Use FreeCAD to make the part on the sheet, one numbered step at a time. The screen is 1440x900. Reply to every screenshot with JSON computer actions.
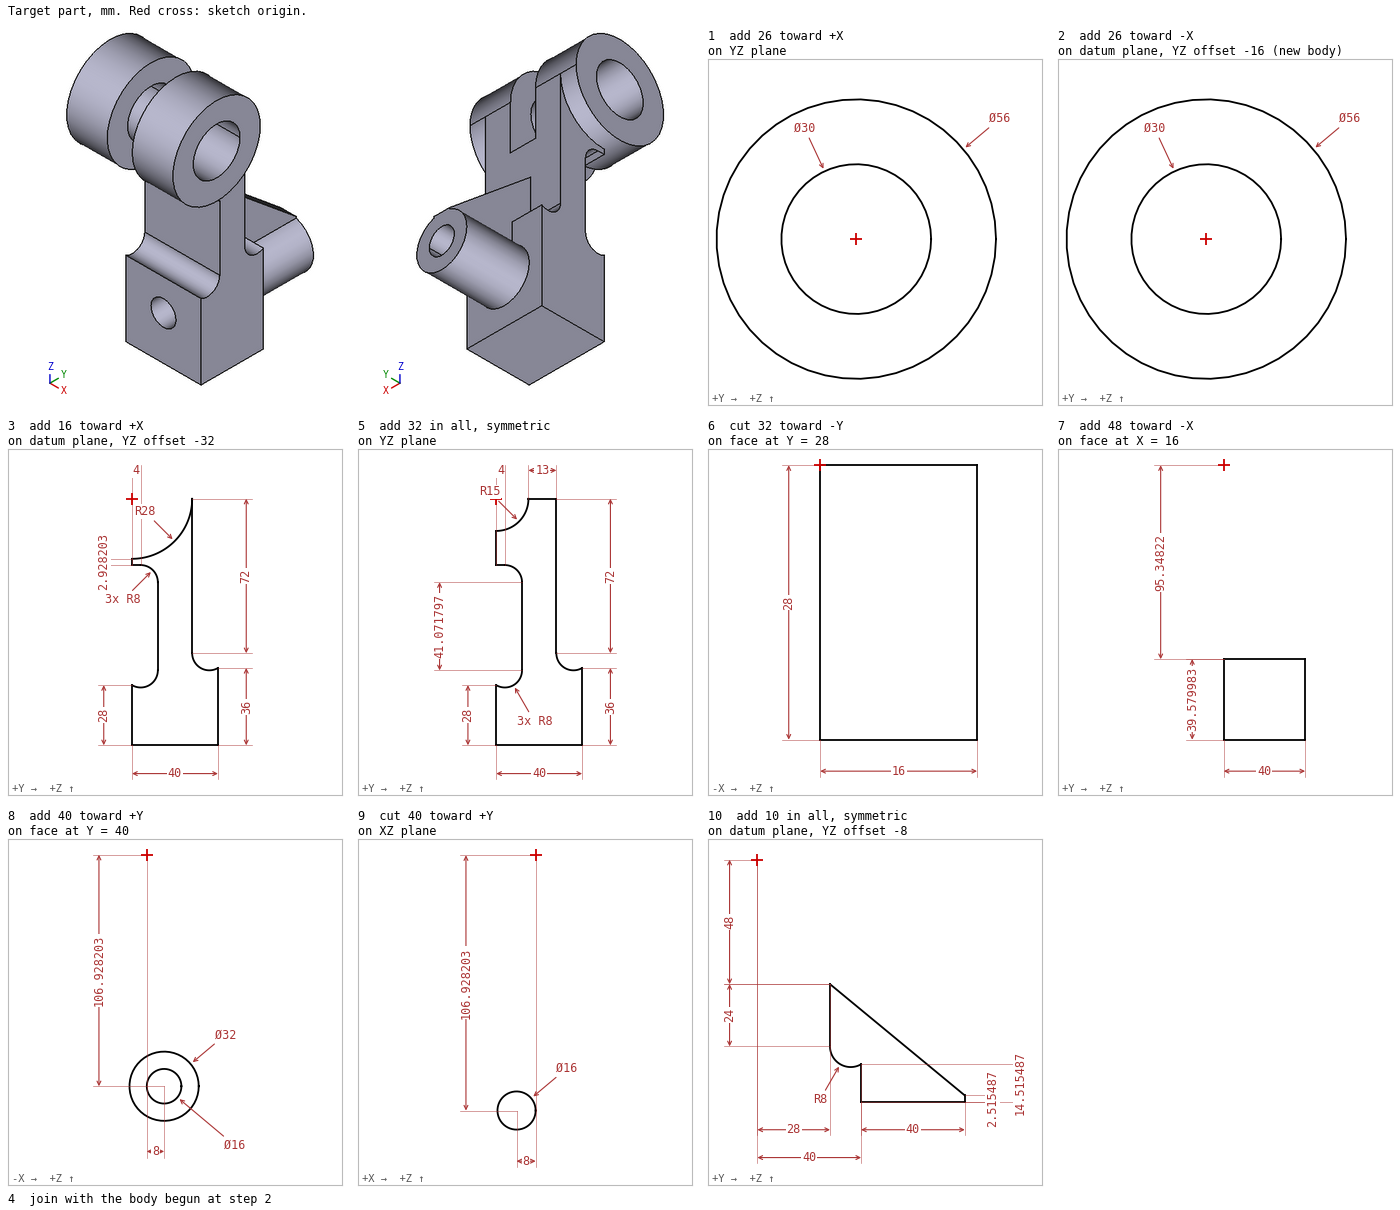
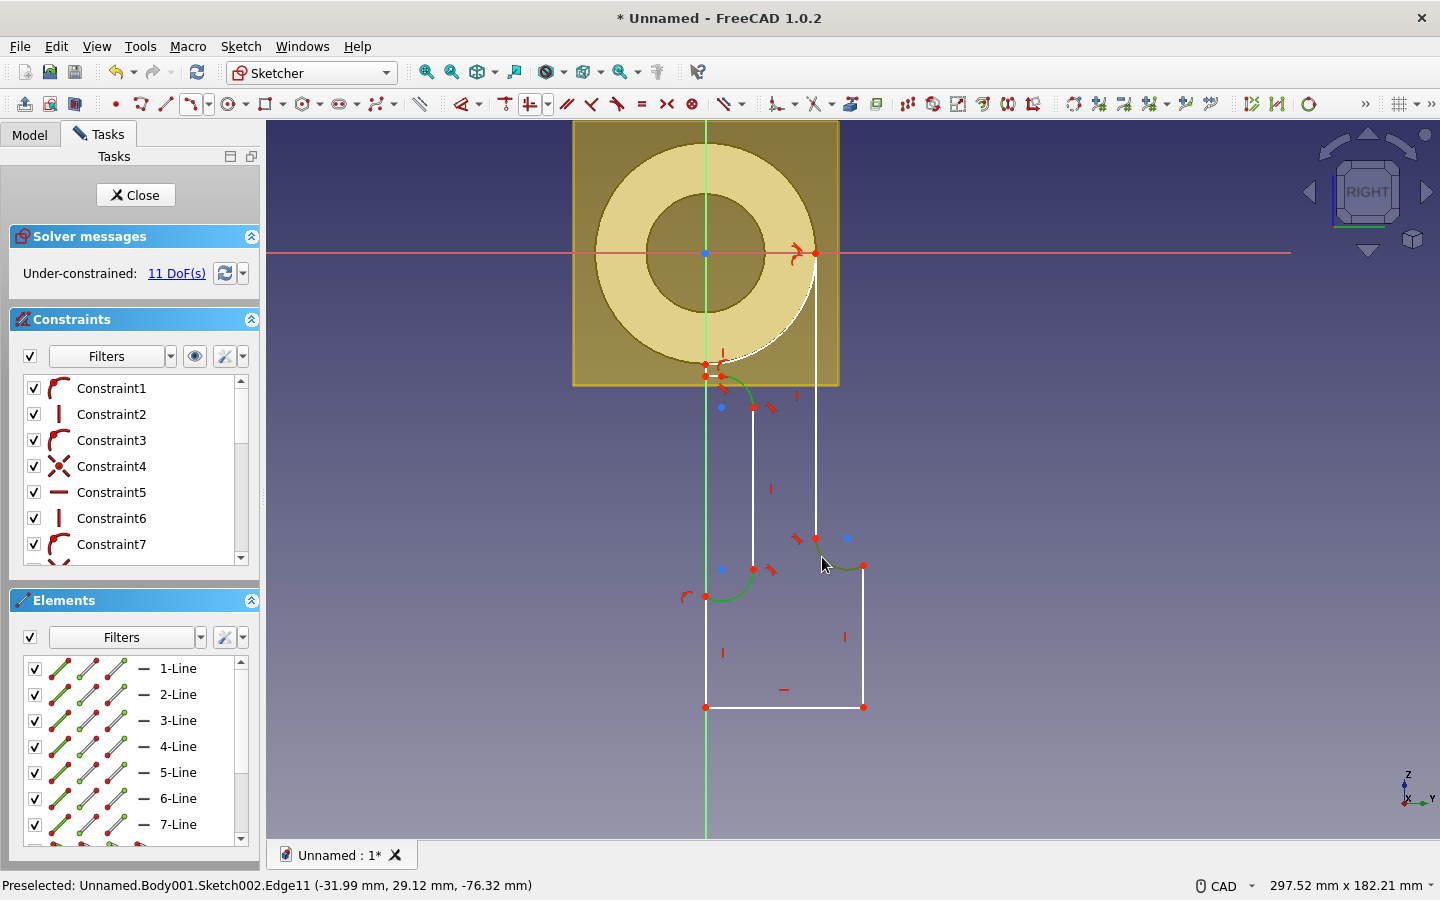
{"action": "key", "text": "e"}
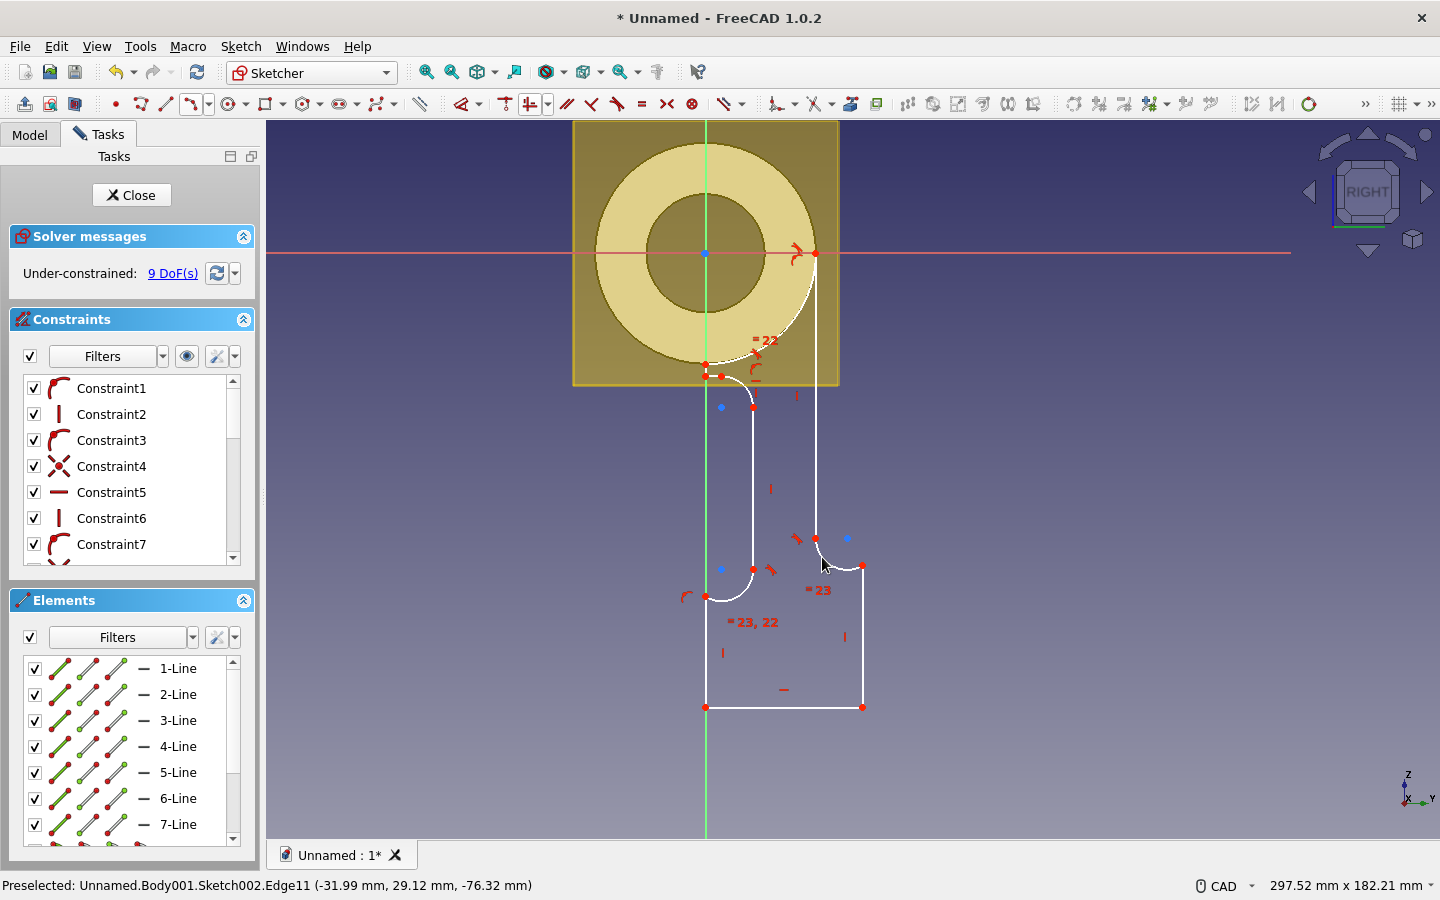
{"action": "left_click", "coordinate": [705, 253]}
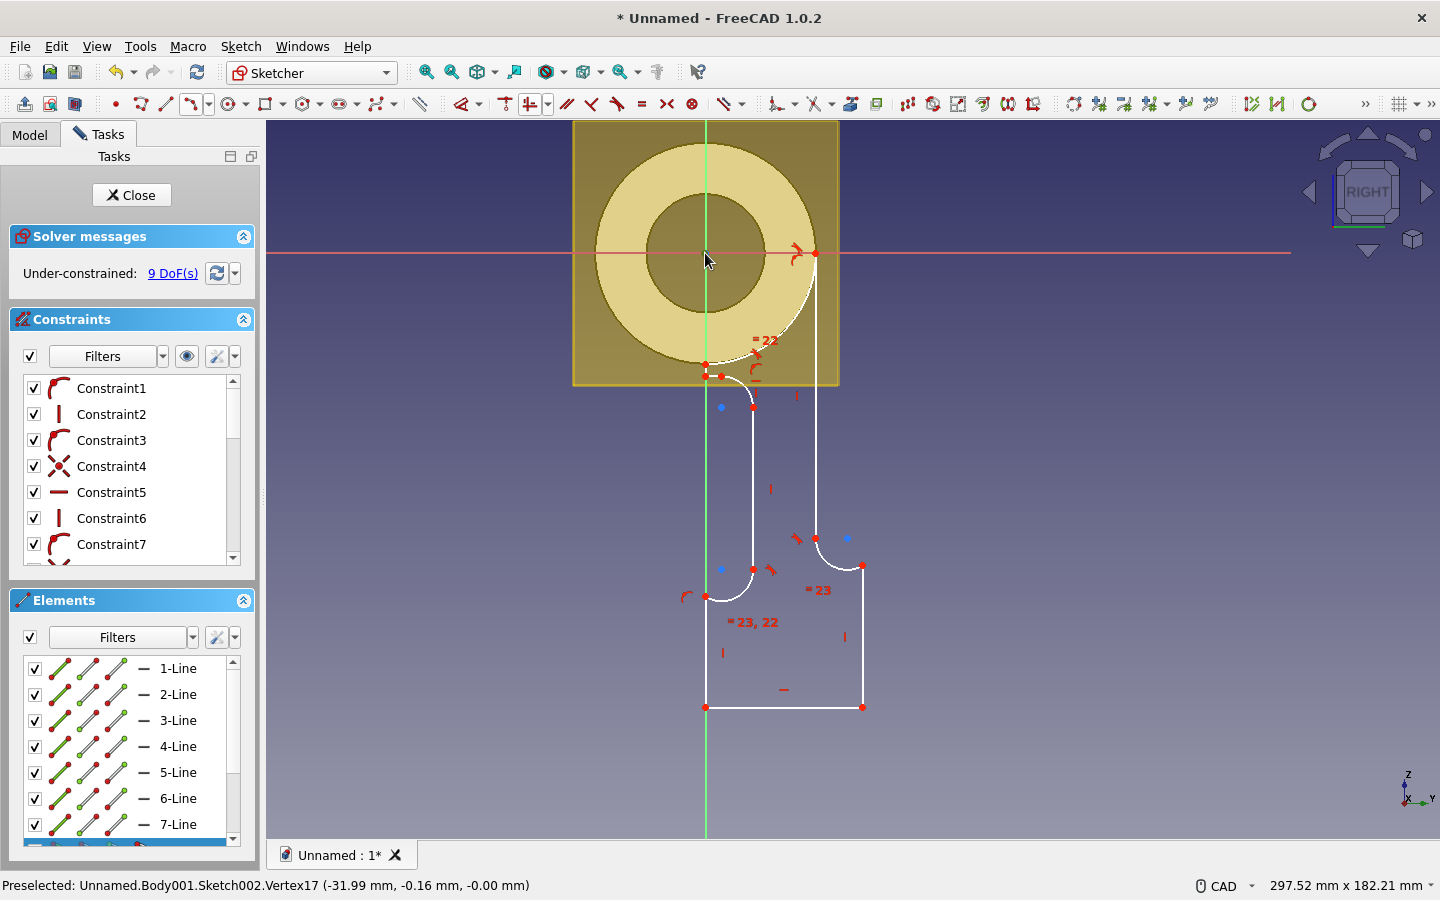
{"action": "left_click", "coordinate": [706, 764]}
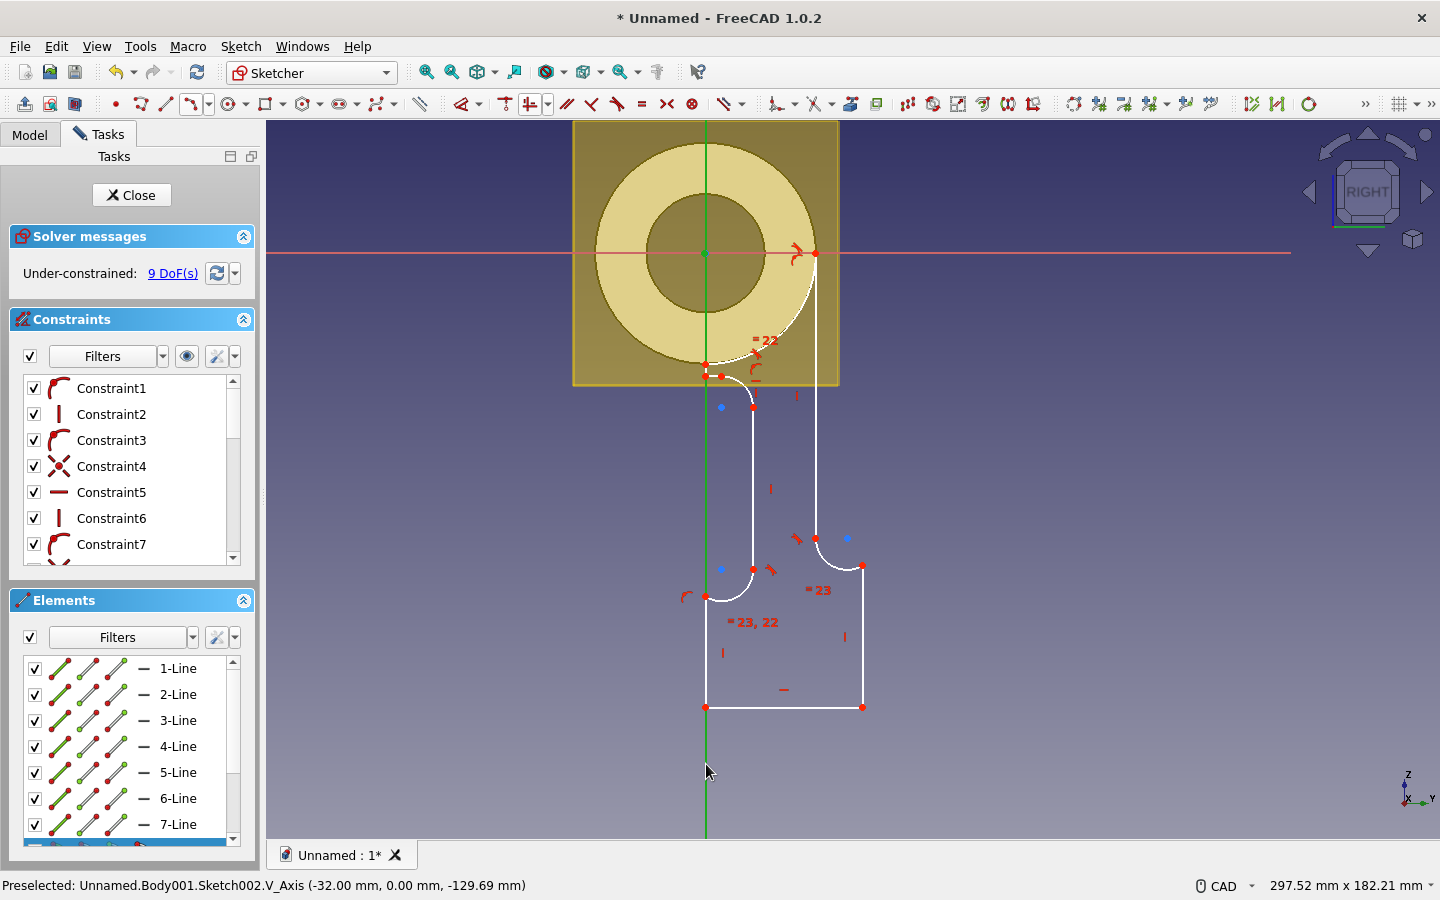
{"action": "key", "text": "c"}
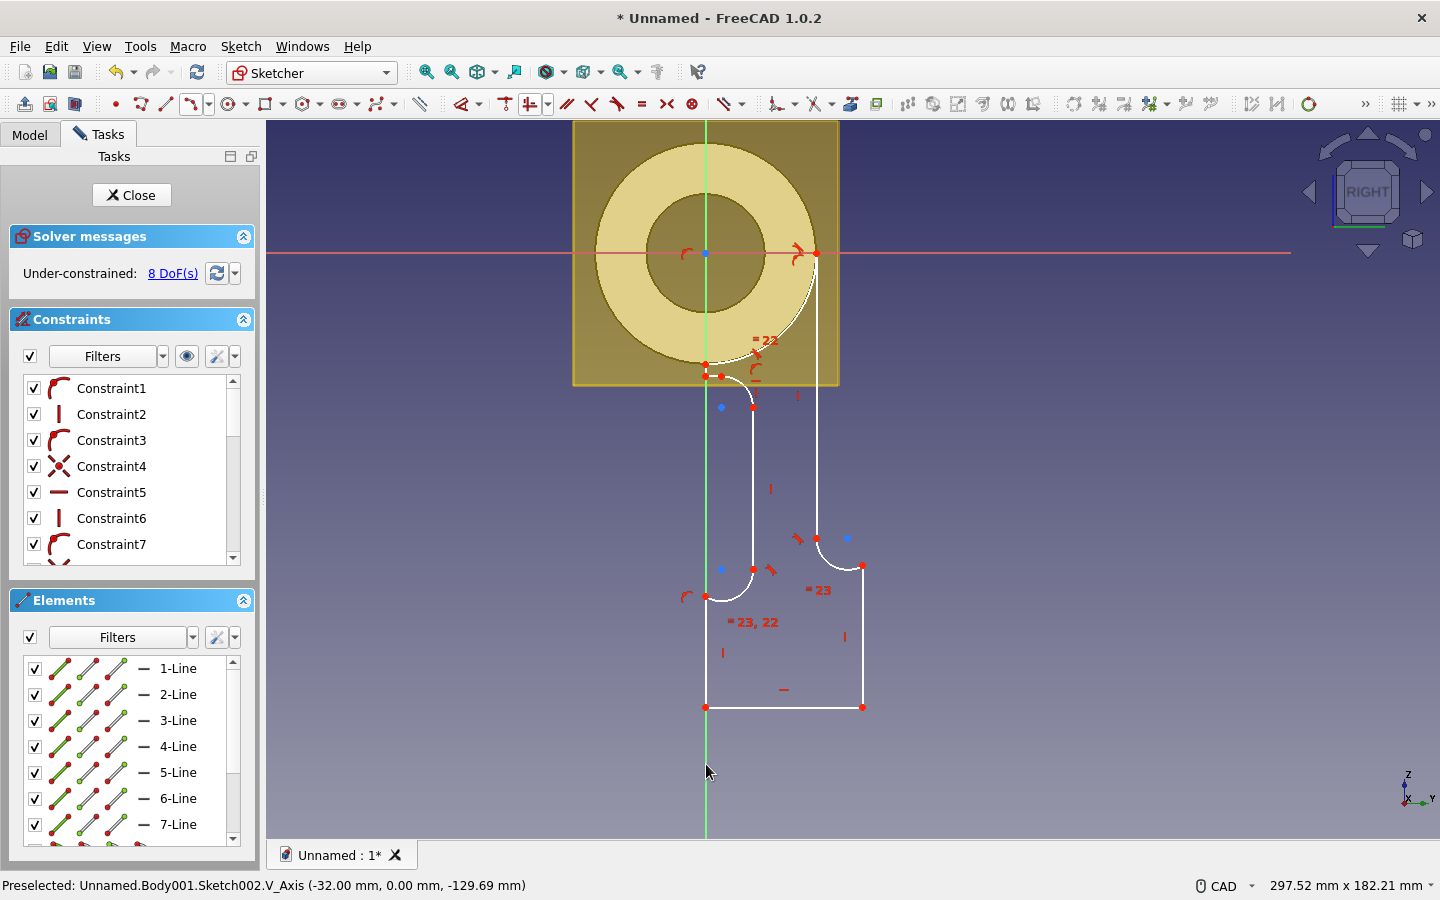
{"action": "left_click", "coordinate": [460, 104]}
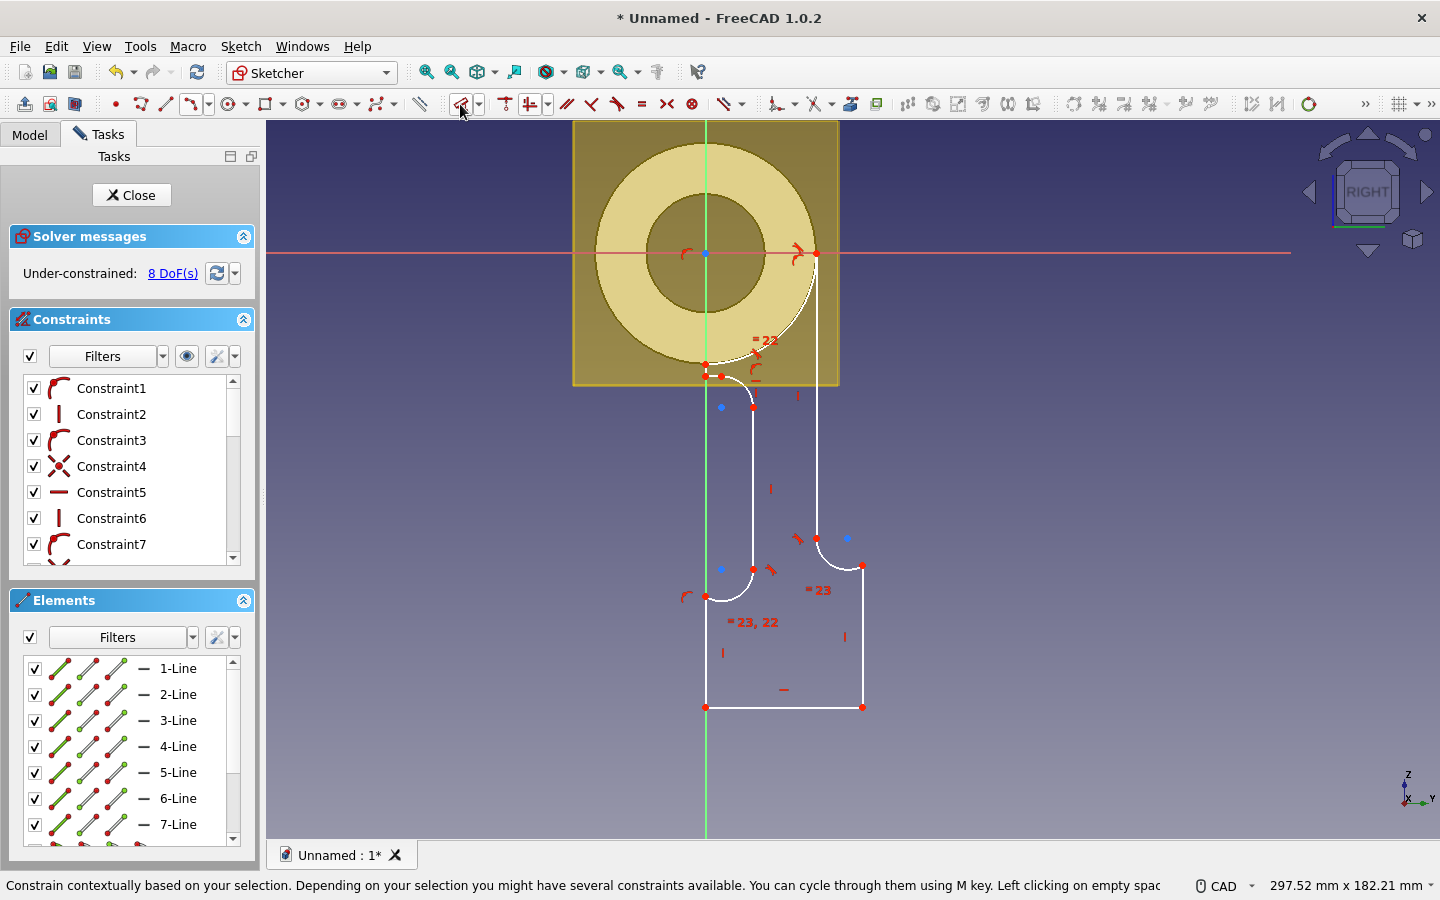
{"action": "left_click", "coordinate": [756, 352]}
{"action": "left_click", "coordinate": [771, 380]}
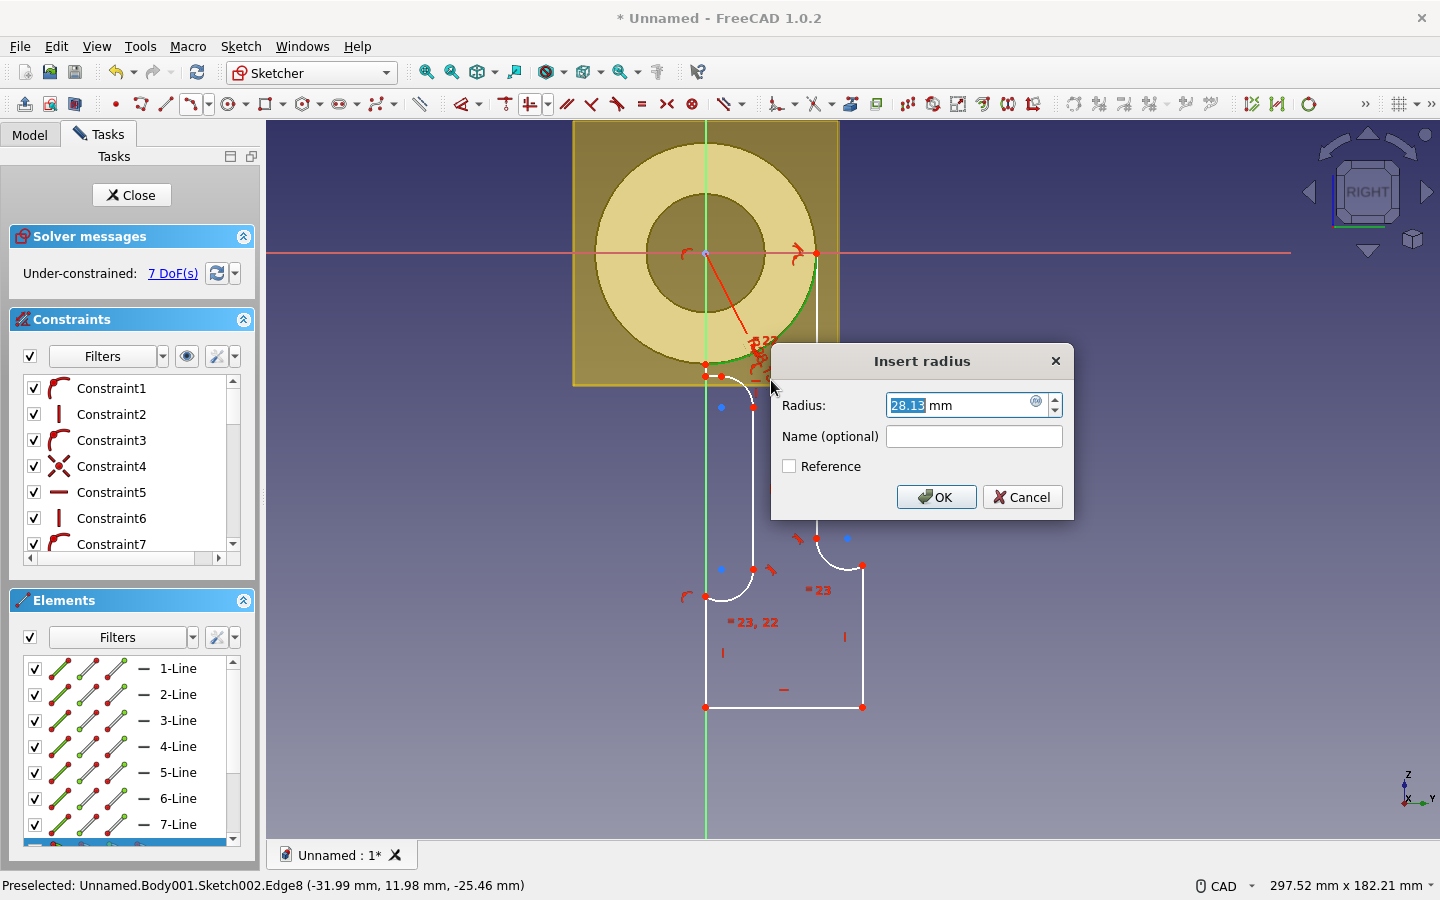
{"action": "type", "text": "28"}
{"action": "key", "text": "Return"}